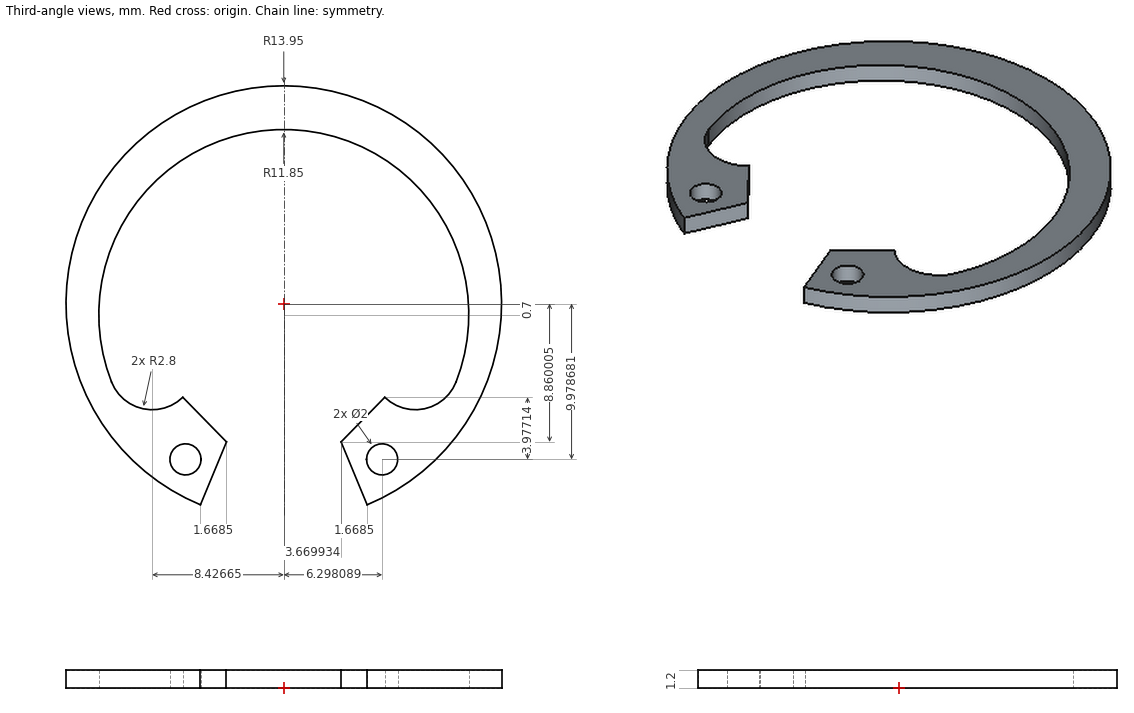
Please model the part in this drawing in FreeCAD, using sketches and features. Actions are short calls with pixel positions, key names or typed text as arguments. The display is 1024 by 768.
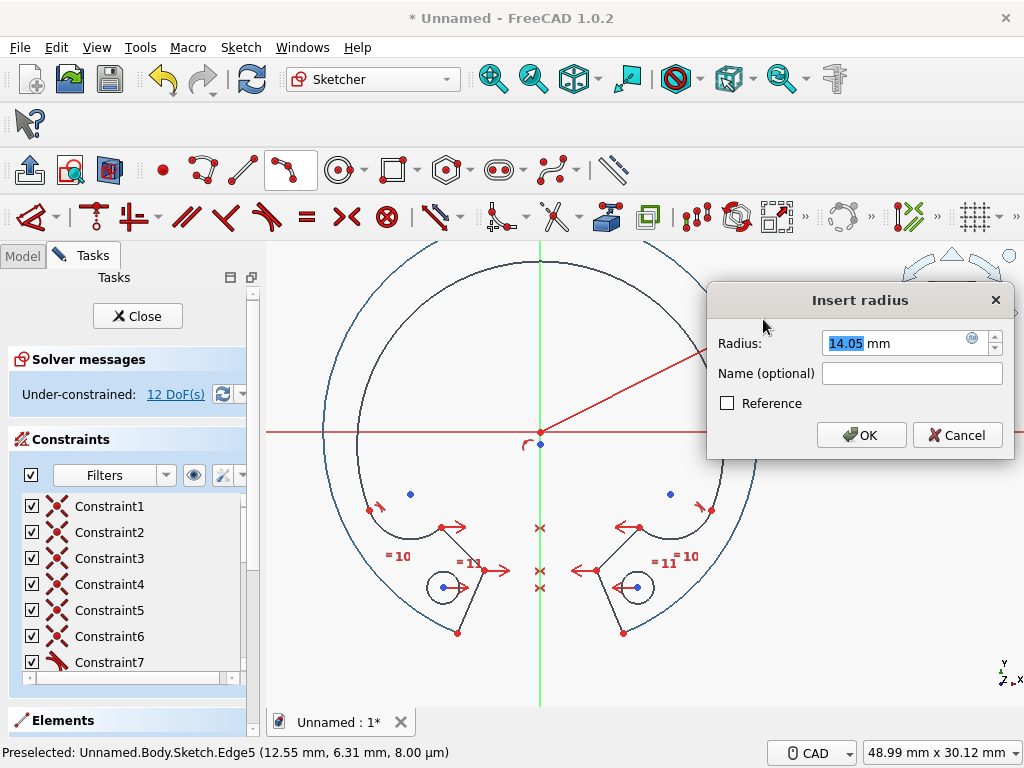
text(13.95)
key(Return)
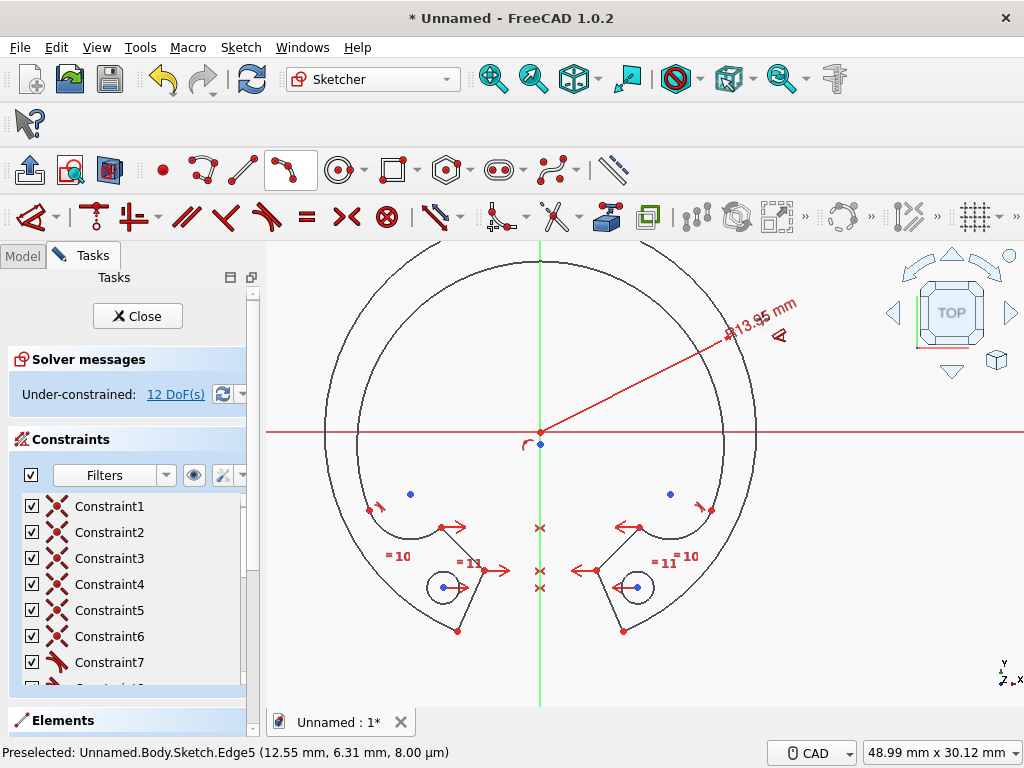
click(385, 531)
click(402, 571)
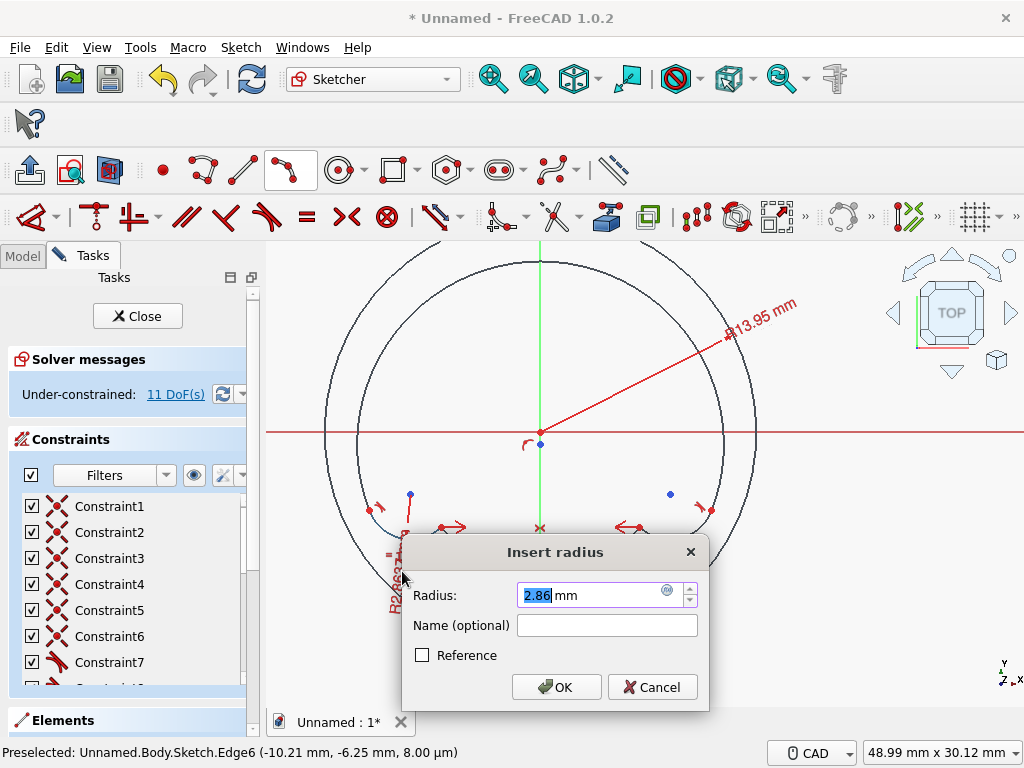
text(2.8)
key(Return)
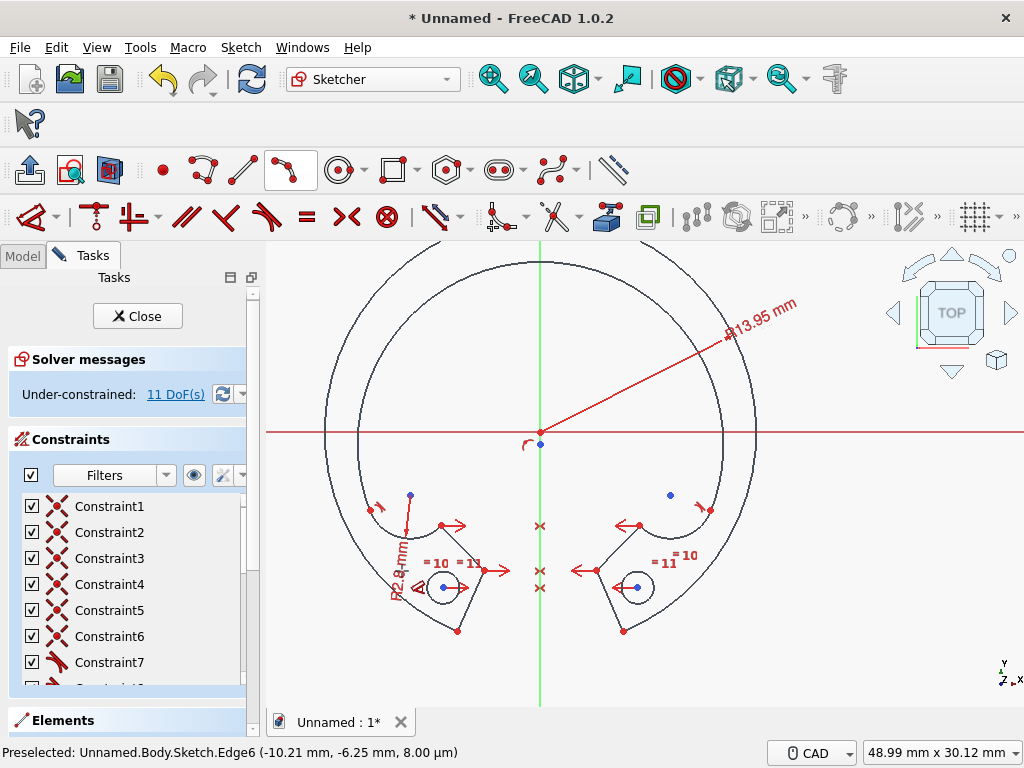
click(669, 314)
click(708, 275)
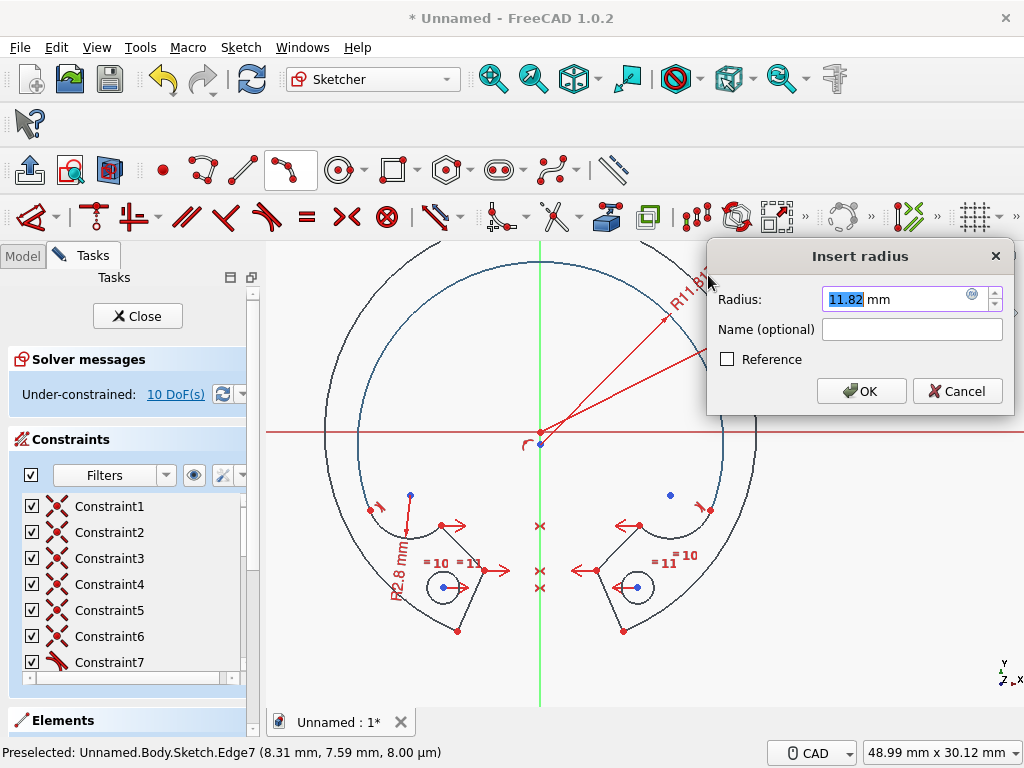
text(11.85)
key(Return)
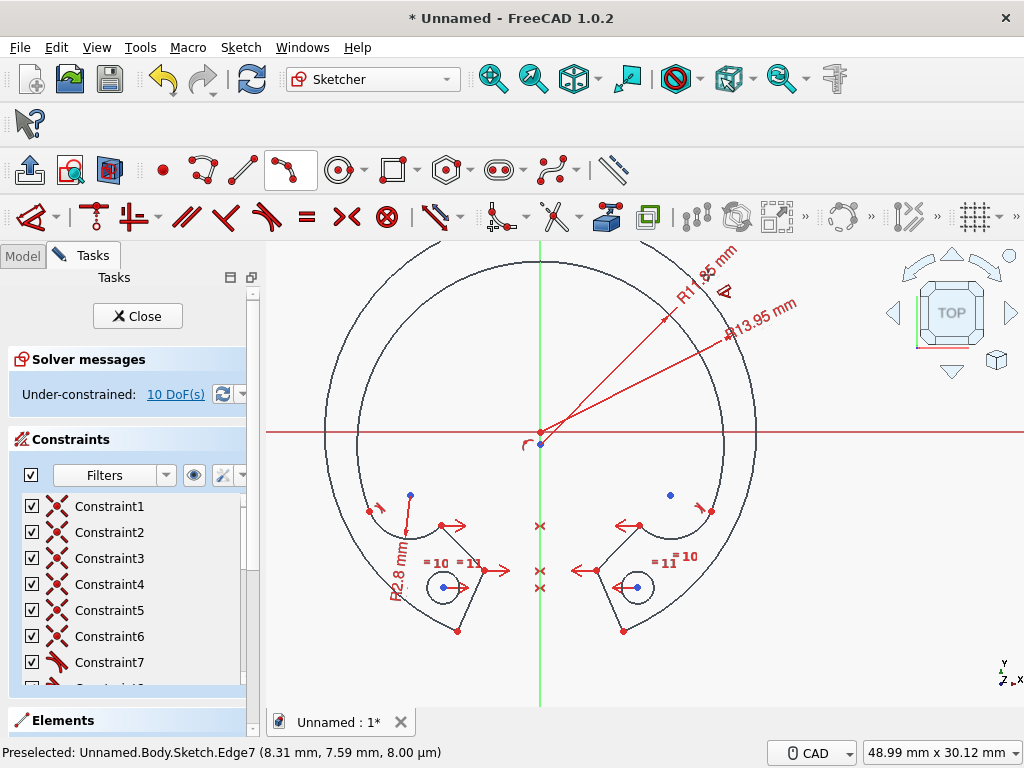
scroll(649, 576, up, 2)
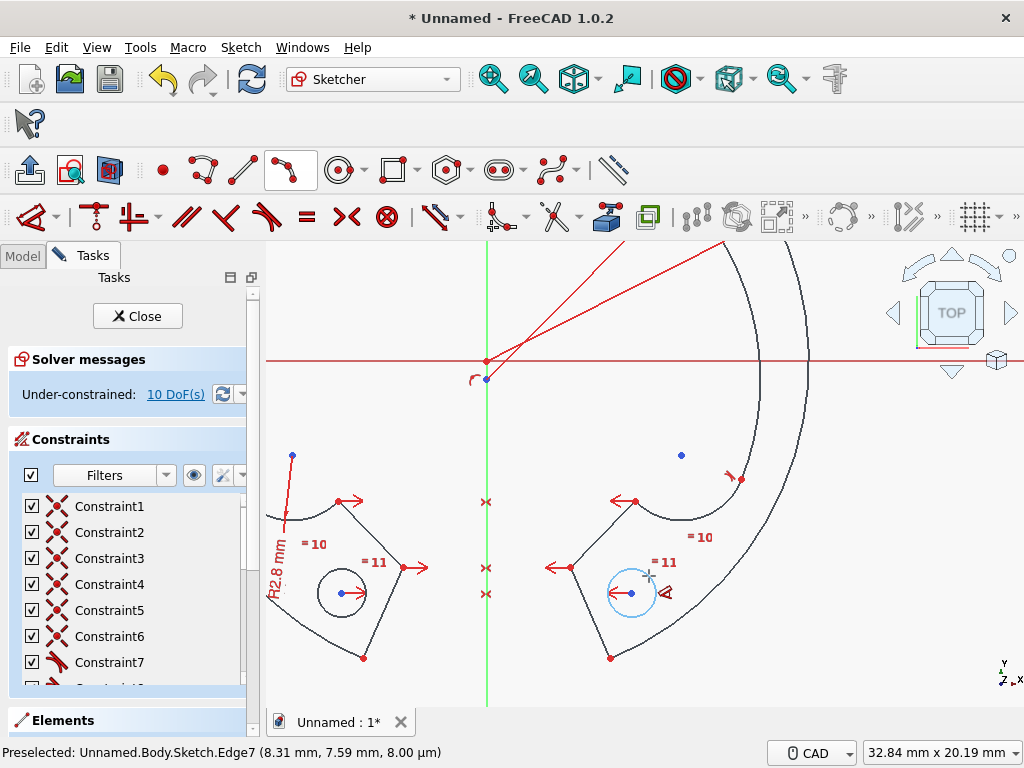
click(649, 576)
click(672, 553)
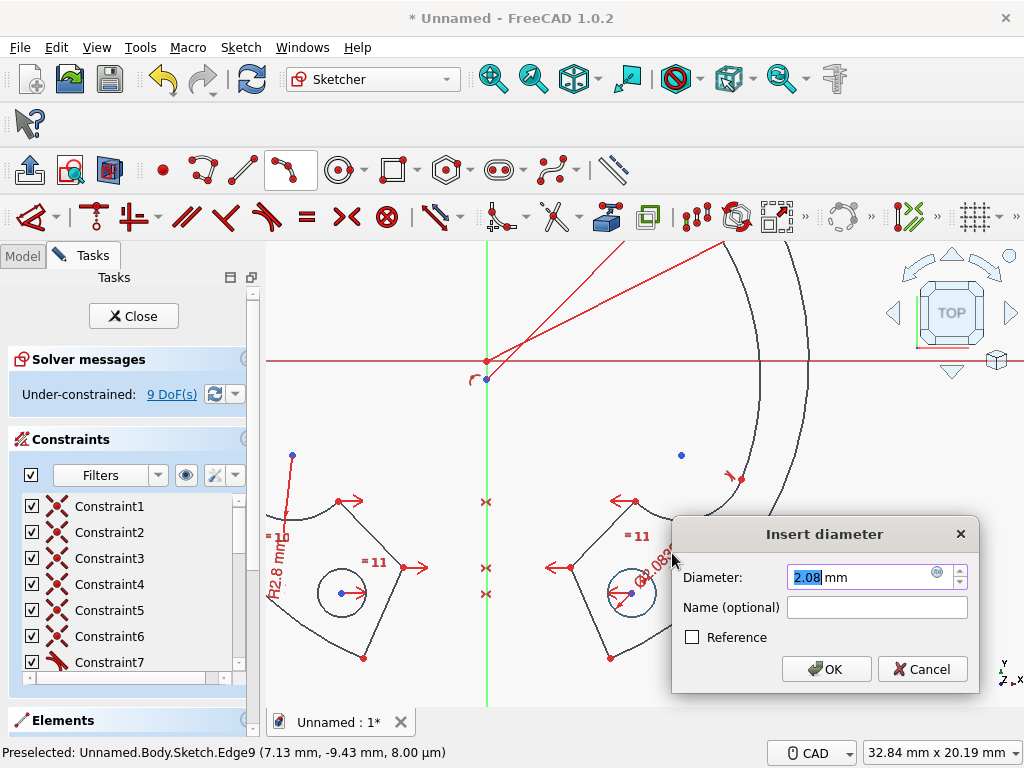
text(2)
key(Return)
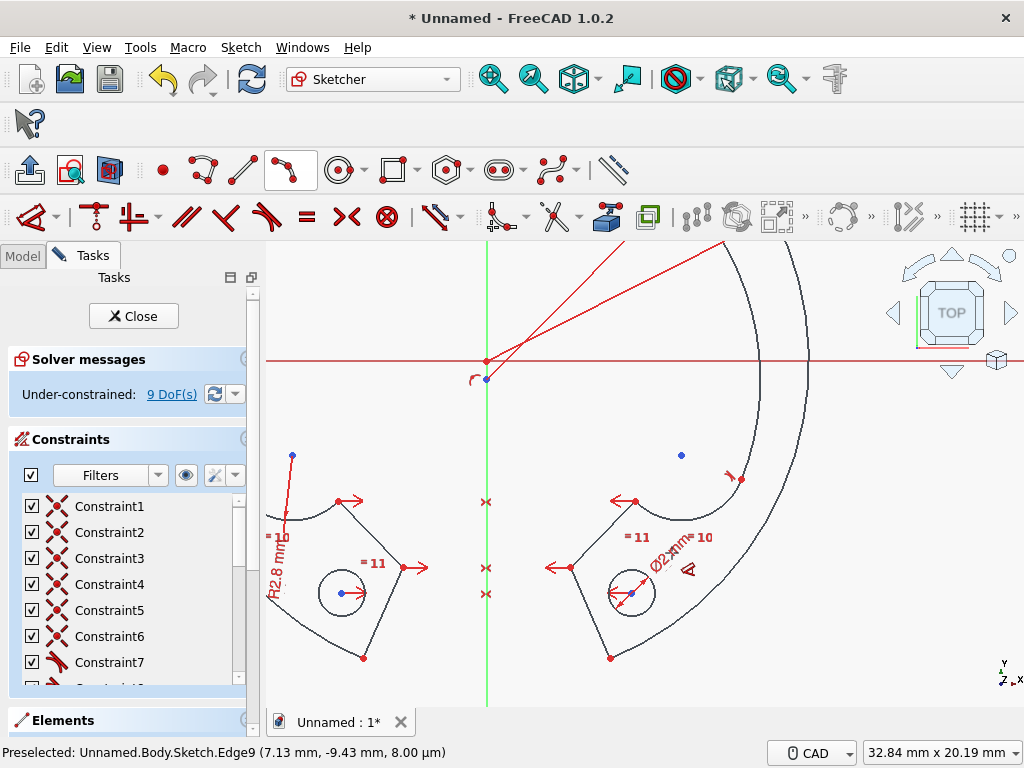
scroll(487, 380, up, 5)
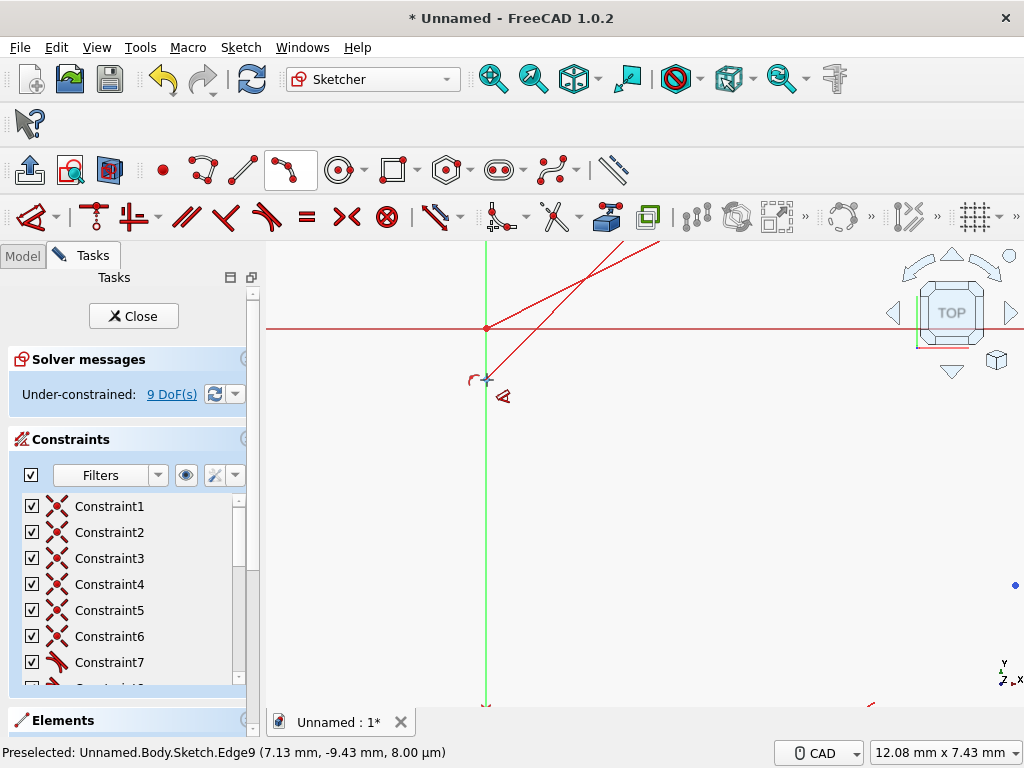
click(486, 379)
click(520, 354)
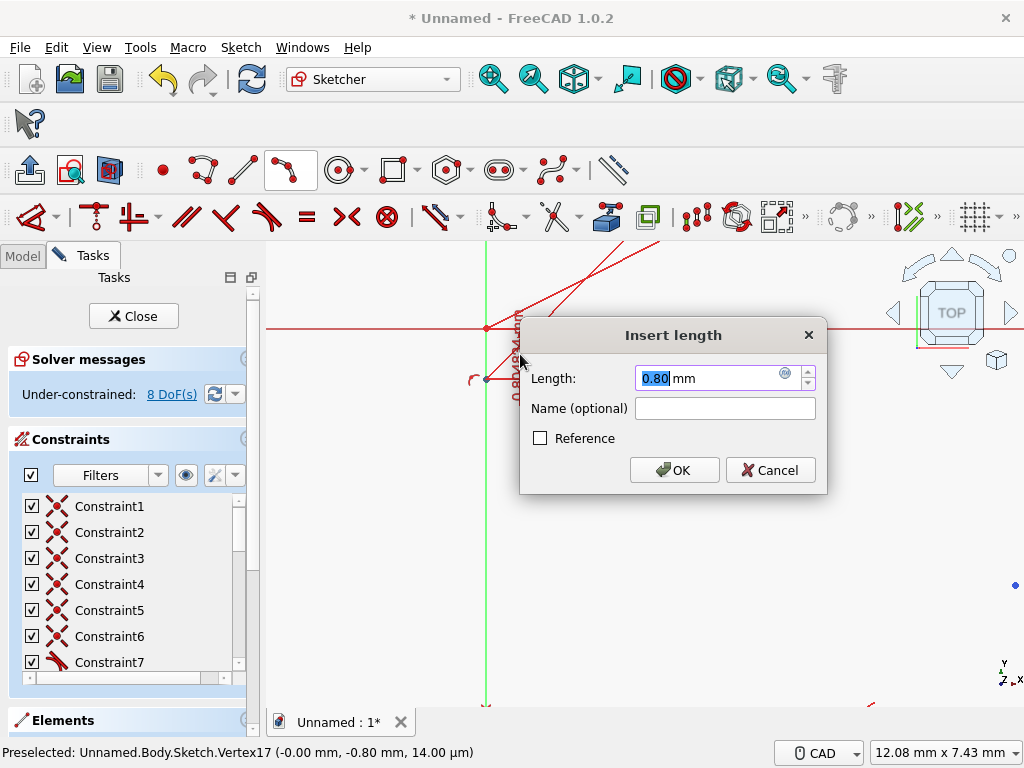
text(0.7)
key(Return)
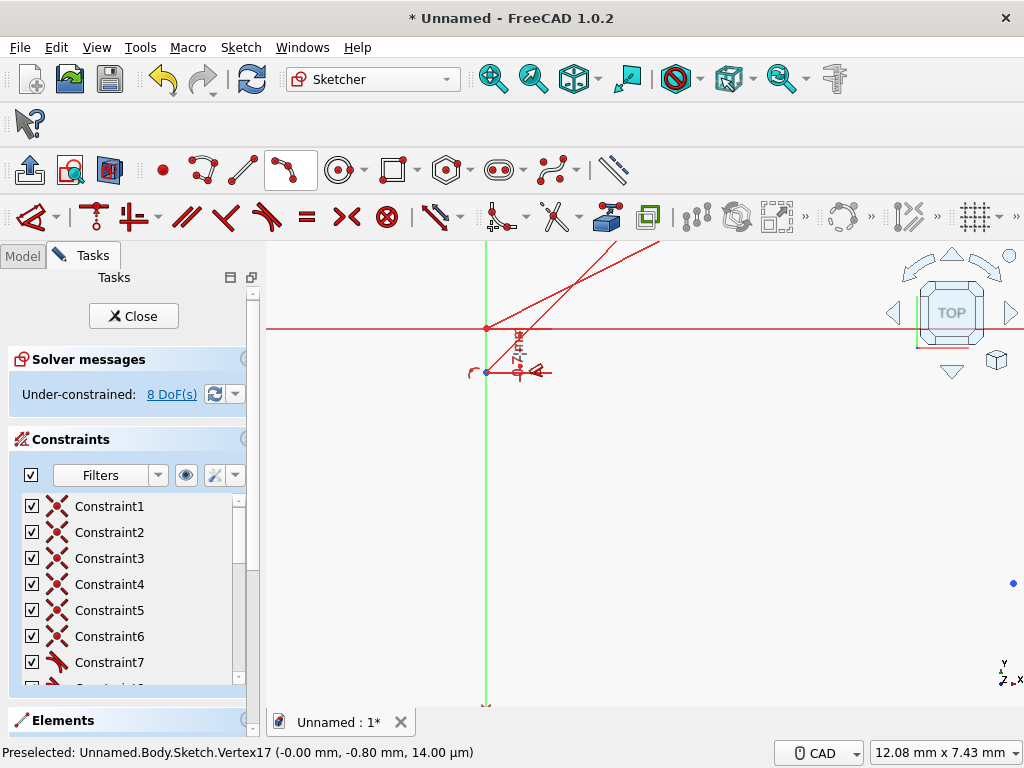
scroll(594, 509, down, 9)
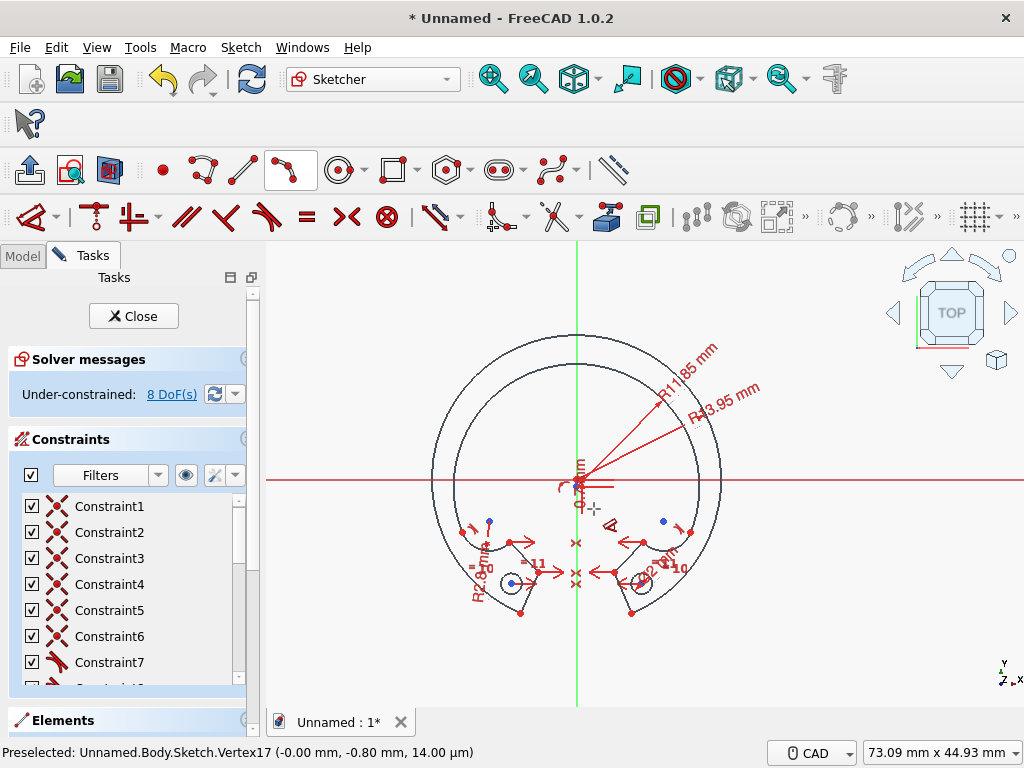
scroll(620, 585, up, 5)